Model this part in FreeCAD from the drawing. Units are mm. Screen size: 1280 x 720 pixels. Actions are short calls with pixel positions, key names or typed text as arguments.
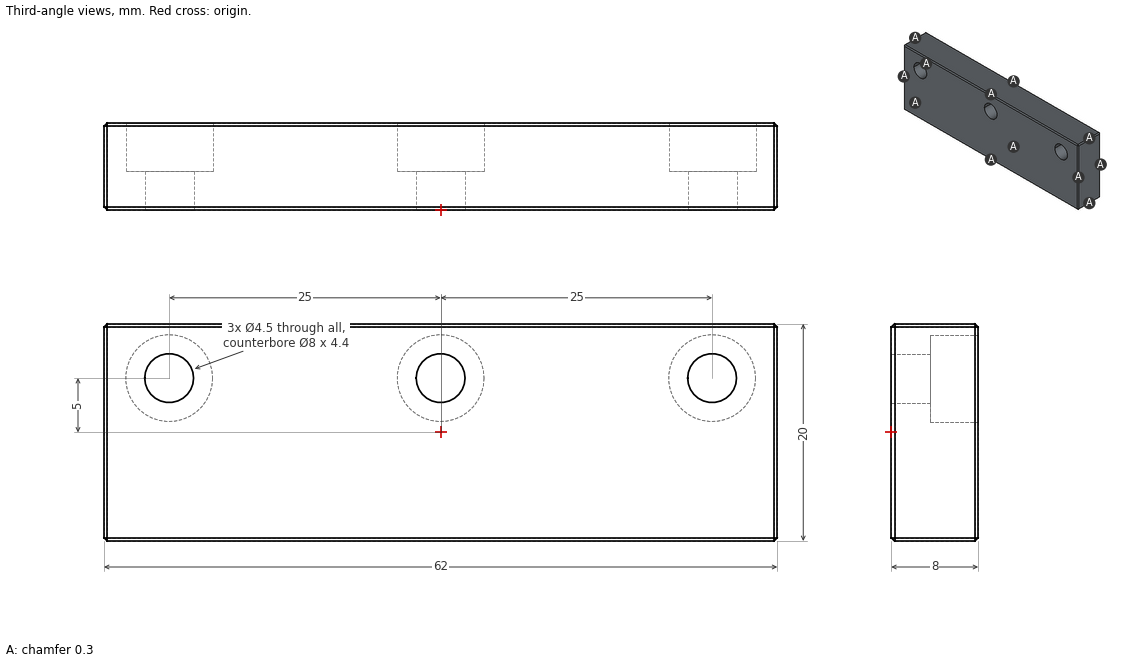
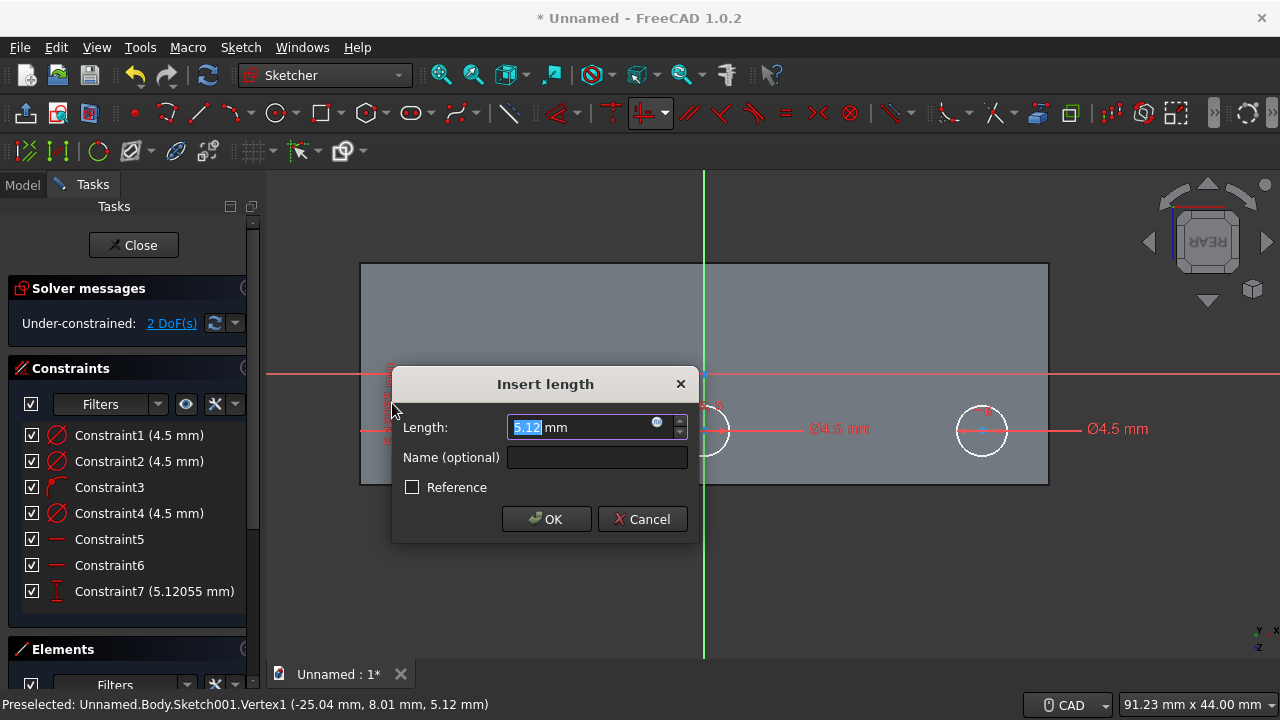
text(5)
key(Return)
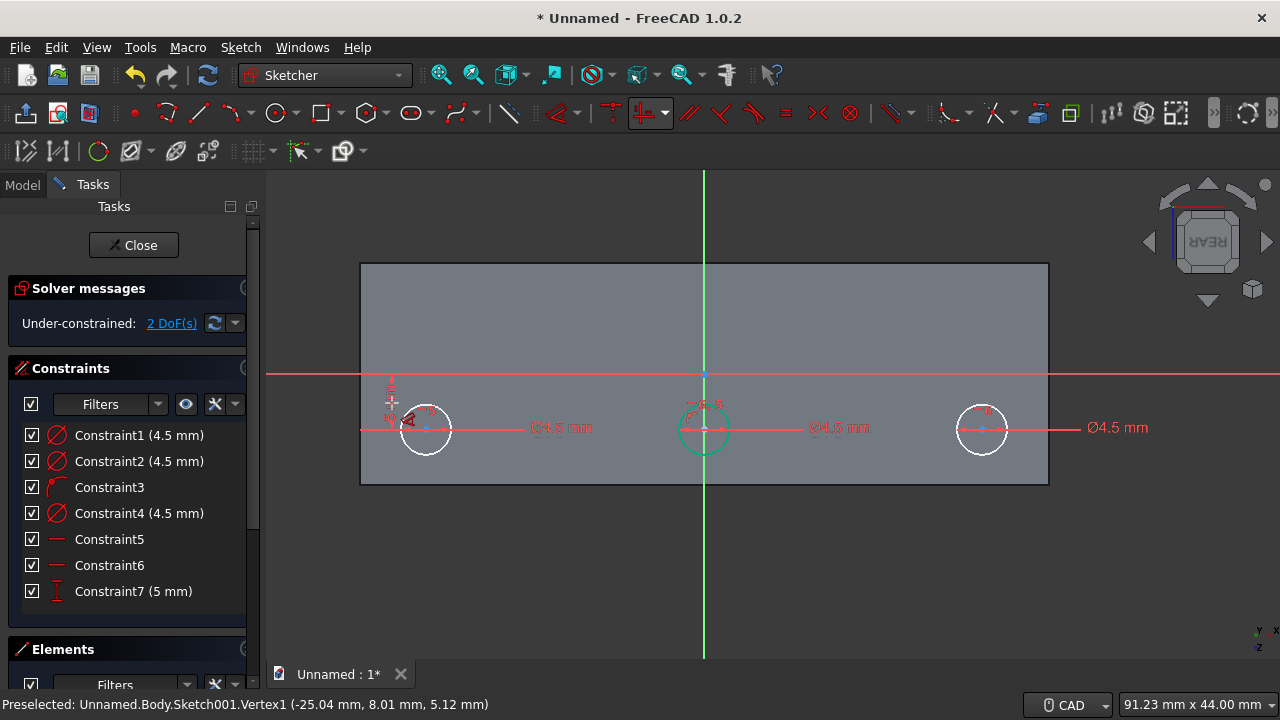
click(426, 430)
click(565, 340)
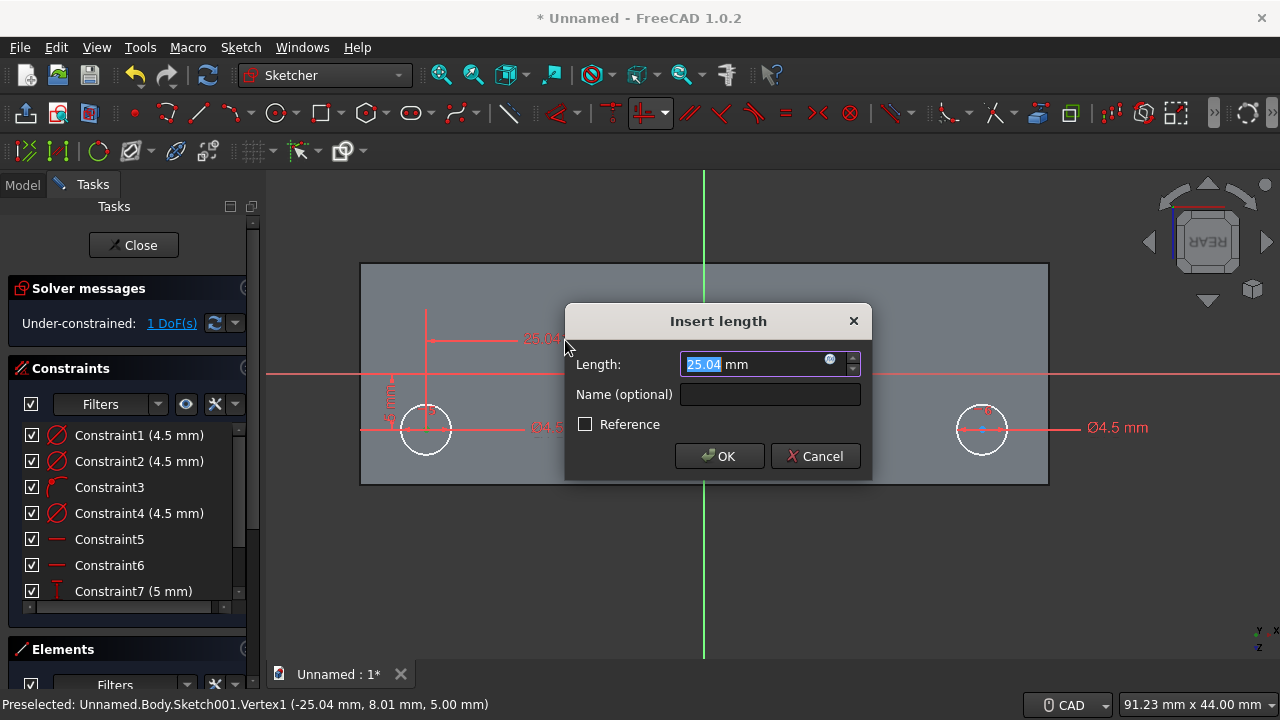
text(25)
key(Return)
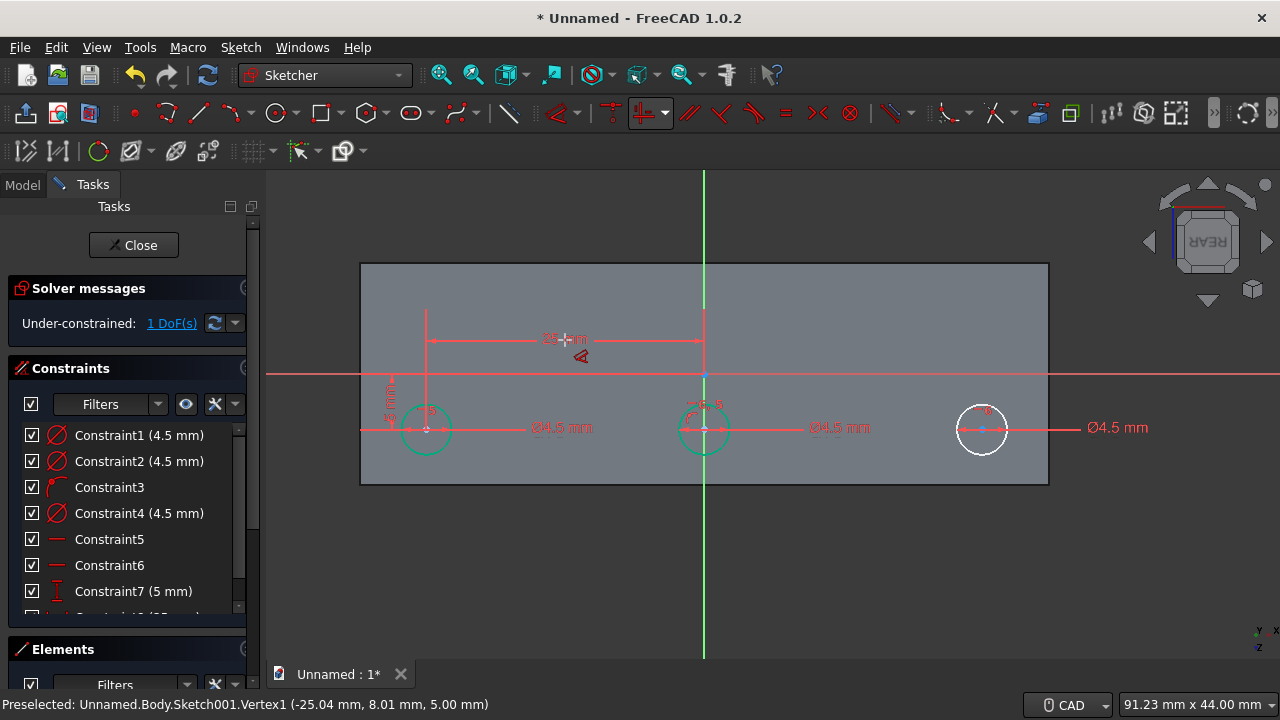
click(982, 430)
click(843, 340)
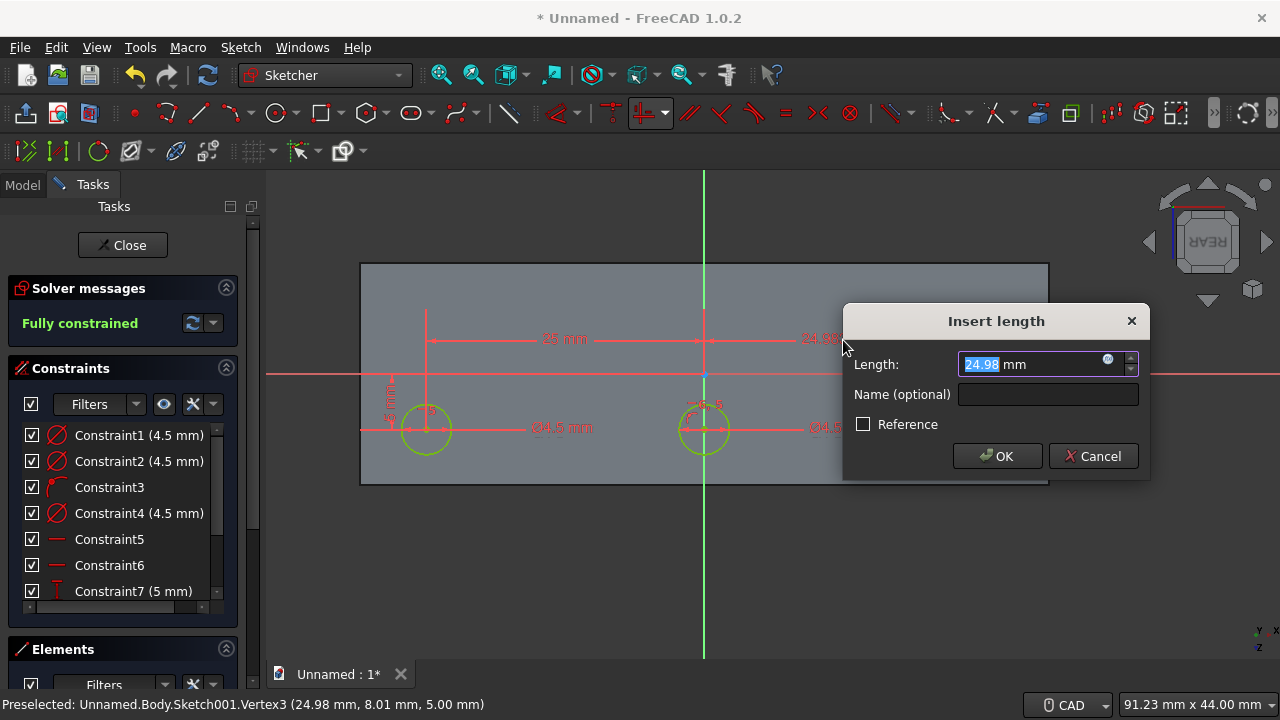
text(25)
key(Return)
key(Escape)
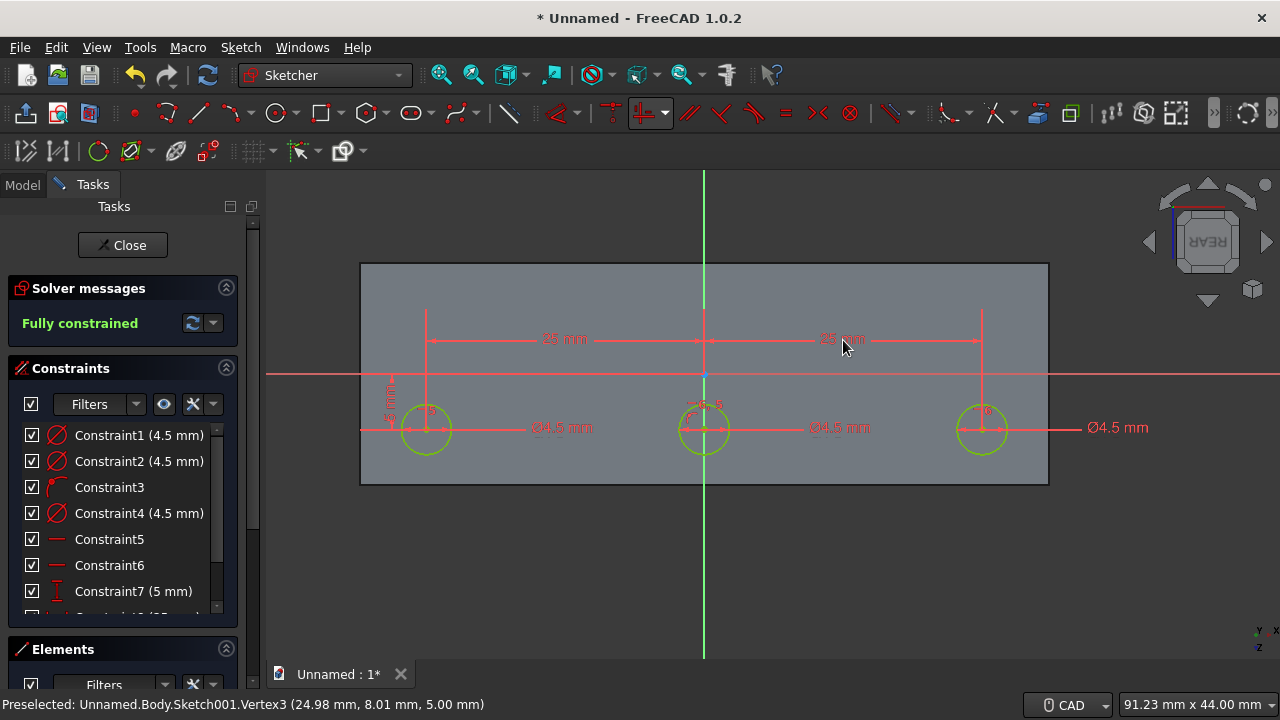
click(123, 245)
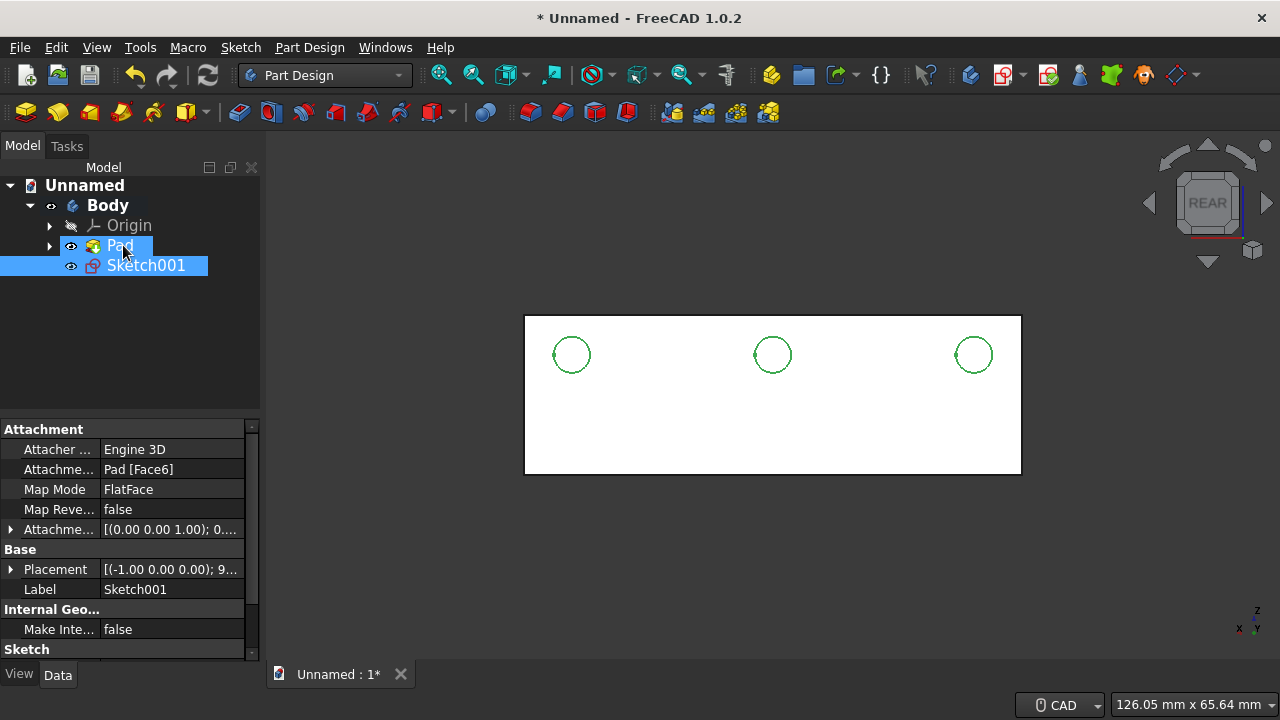
click(272, 112)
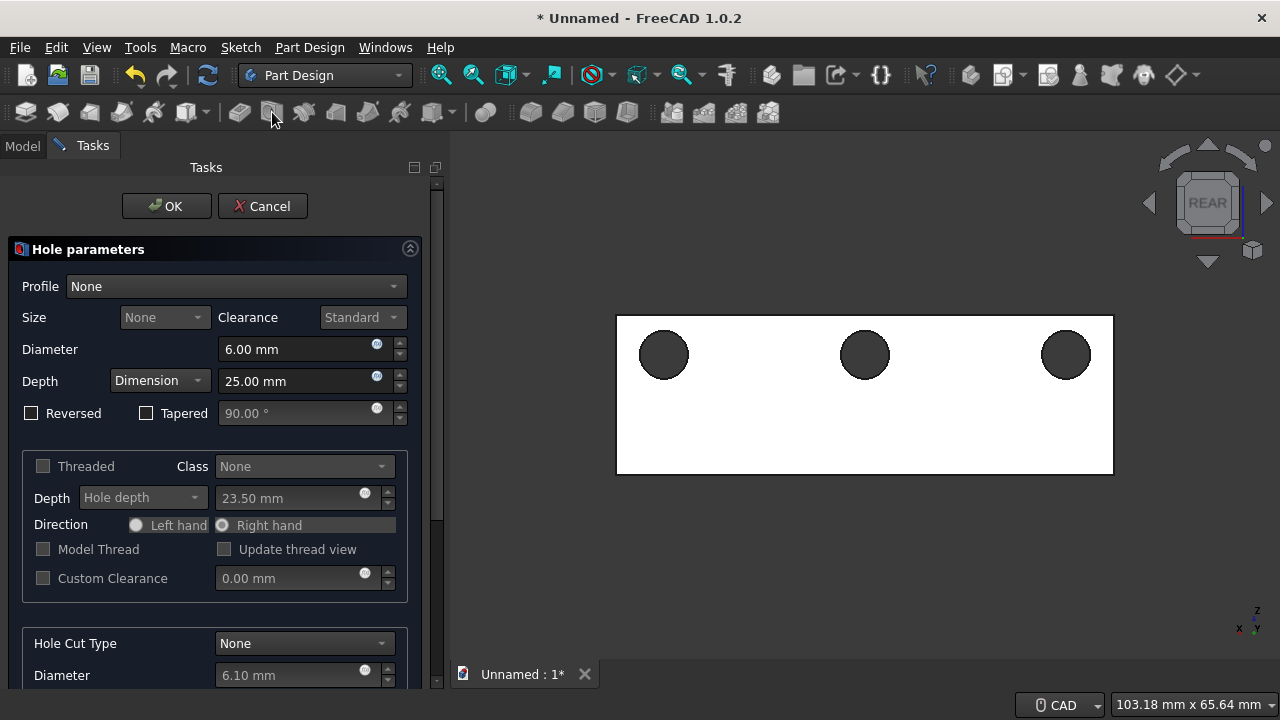
triple_click(305, 349)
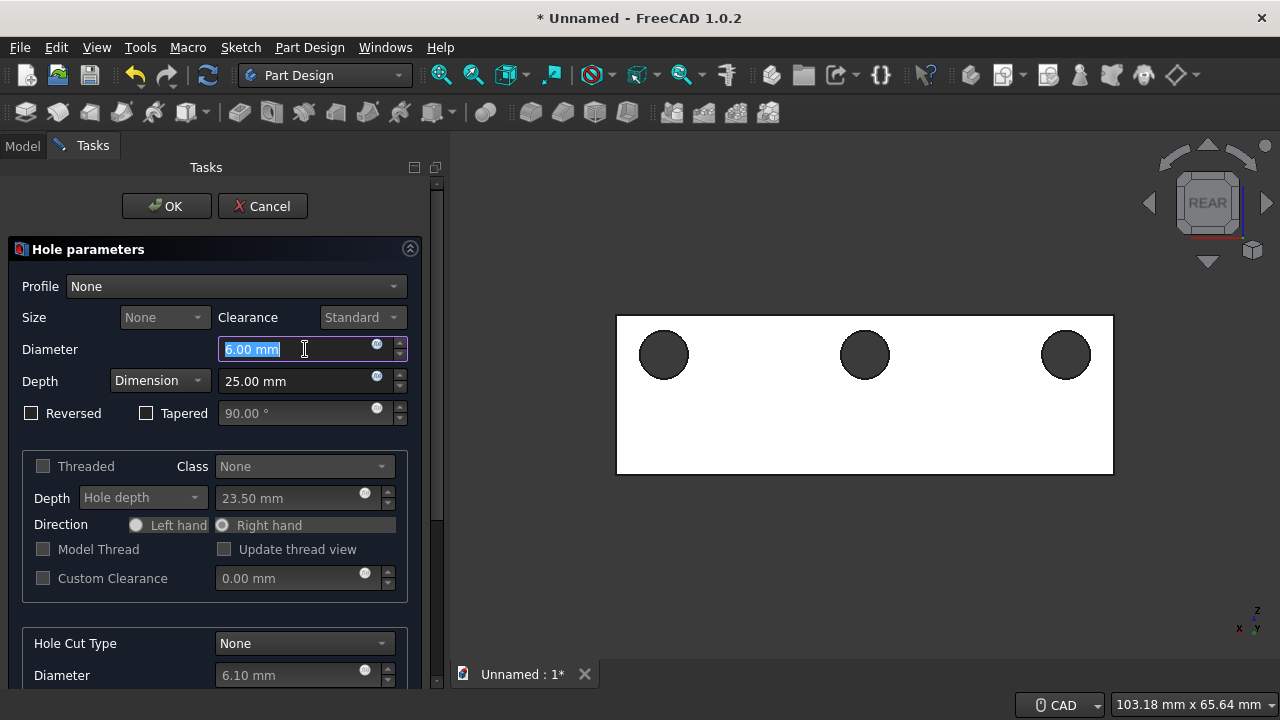
text(4.5)
key(Tab)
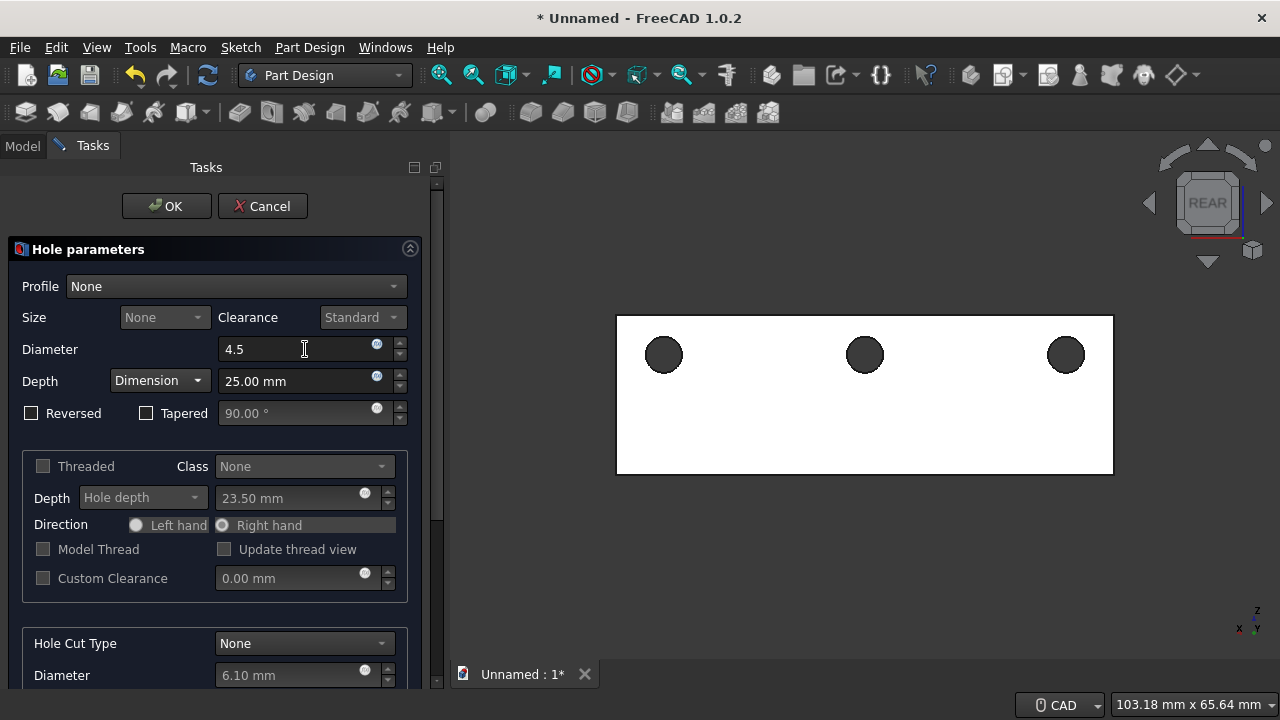
click(161, 380)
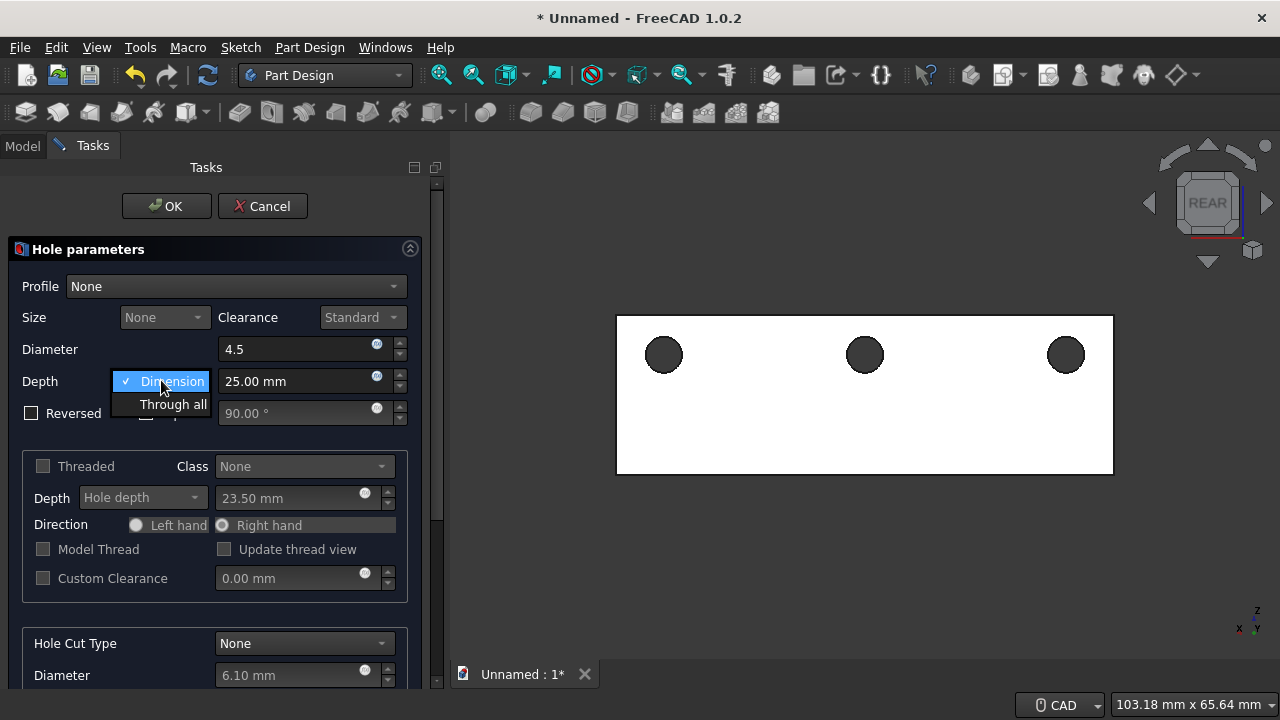
click(160, 404)